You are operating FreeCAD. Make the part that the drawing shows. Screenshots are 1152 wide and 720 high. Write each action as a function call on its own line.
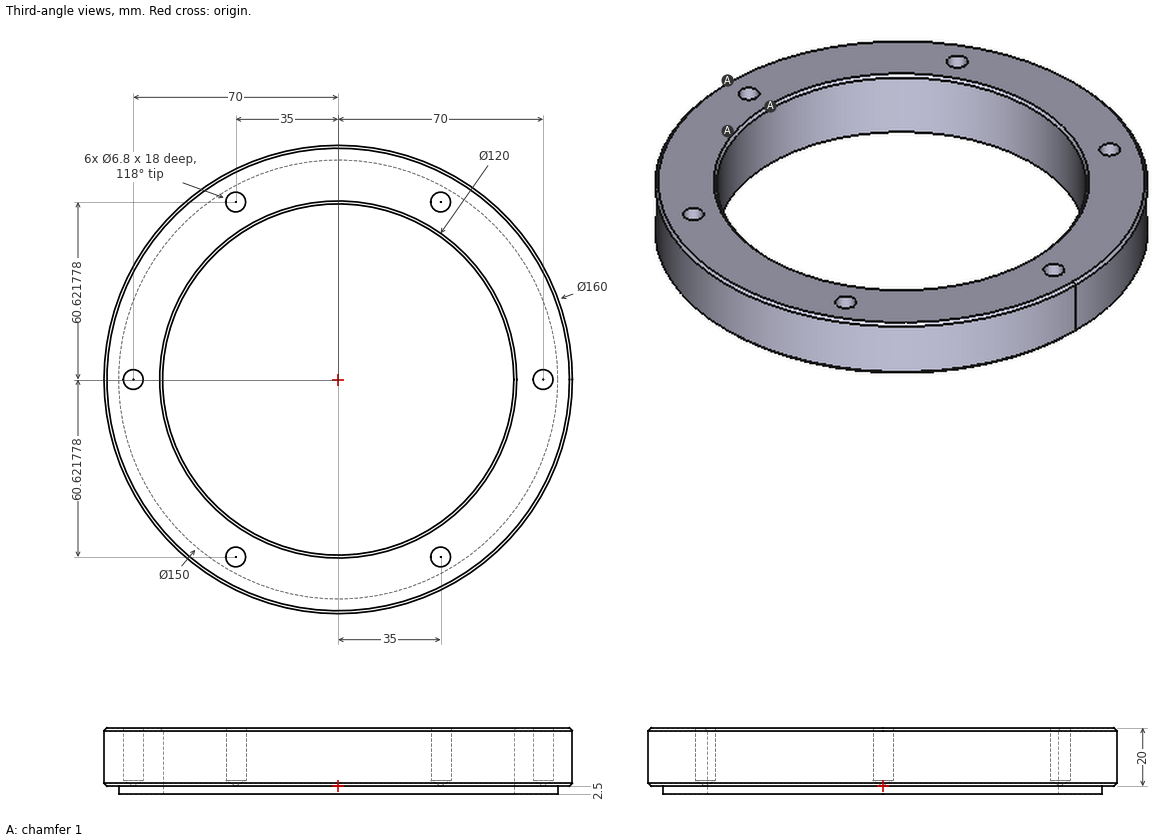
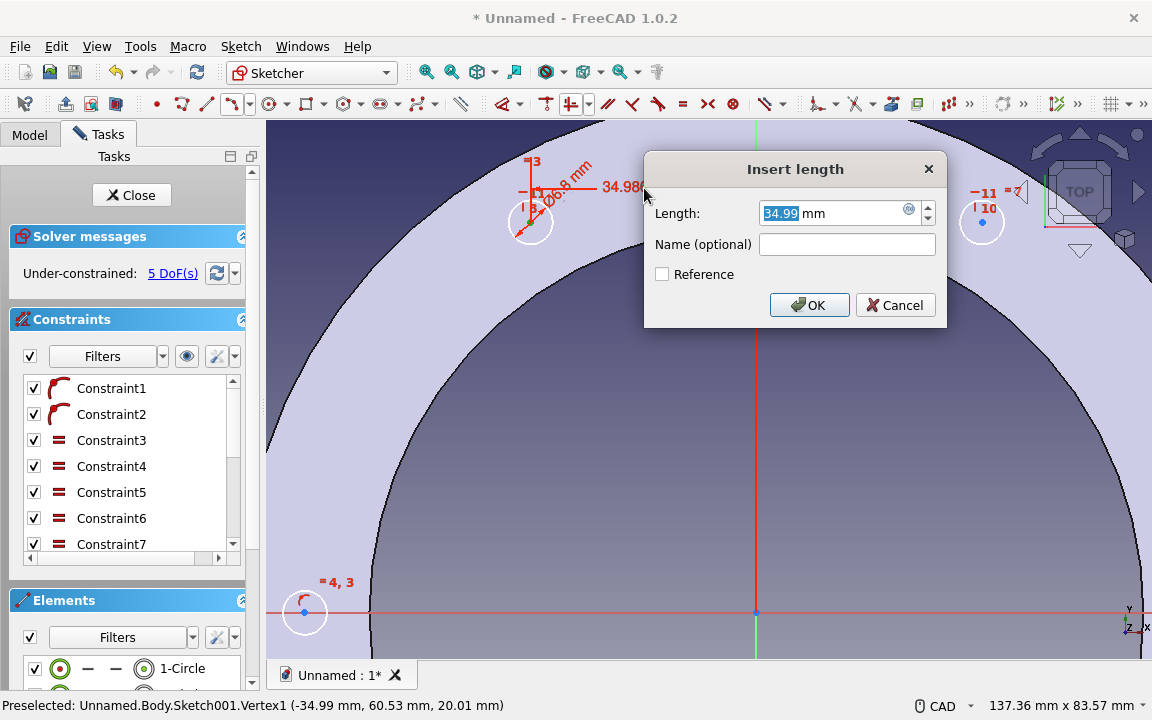
text(35)
key(Return)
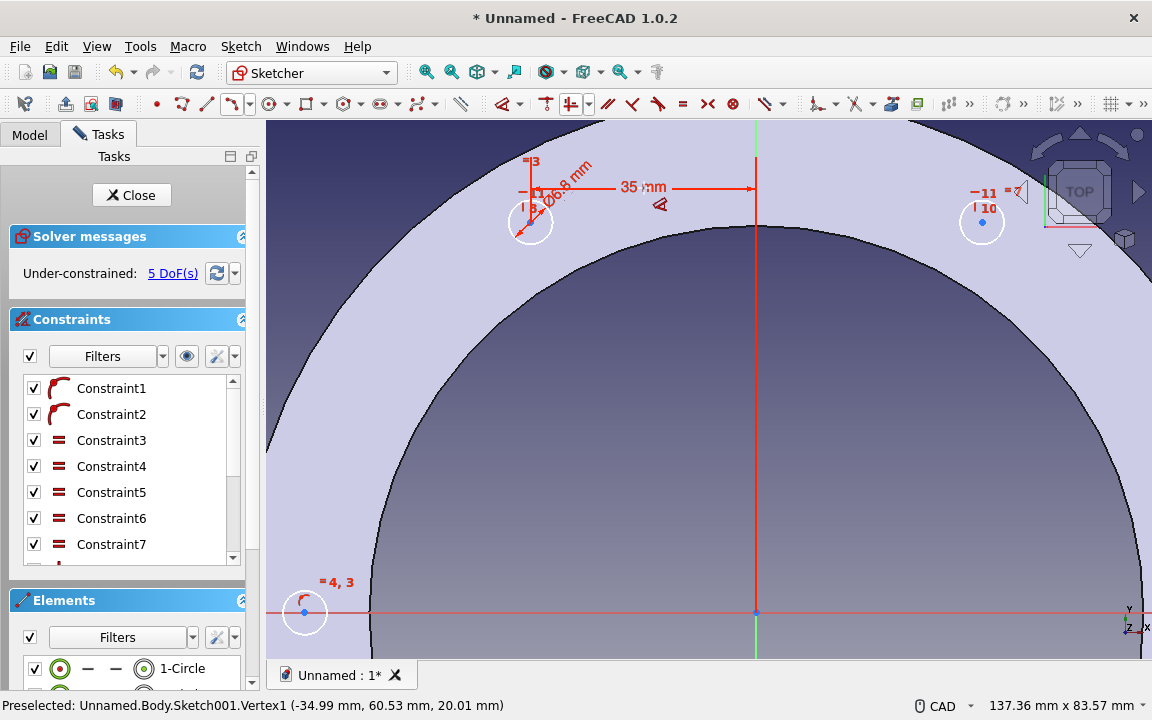
click(305, 613)
click(531, 579)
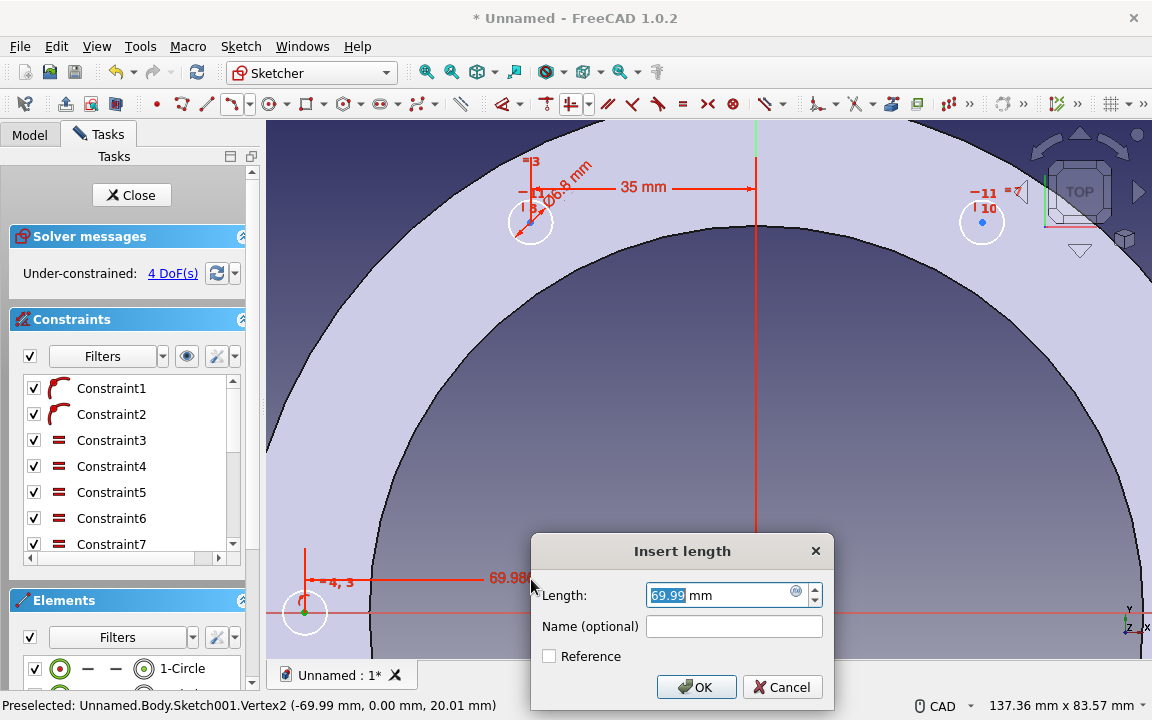
text(70)
key(Return)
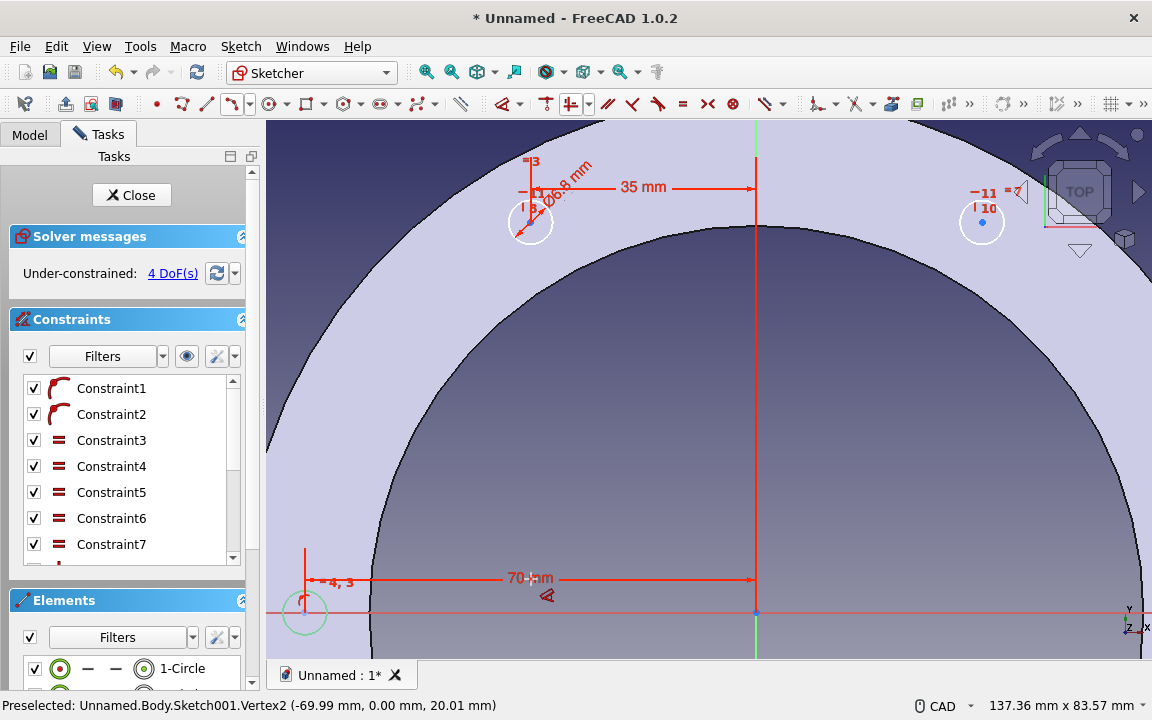
scroll(546, 207, down, 4)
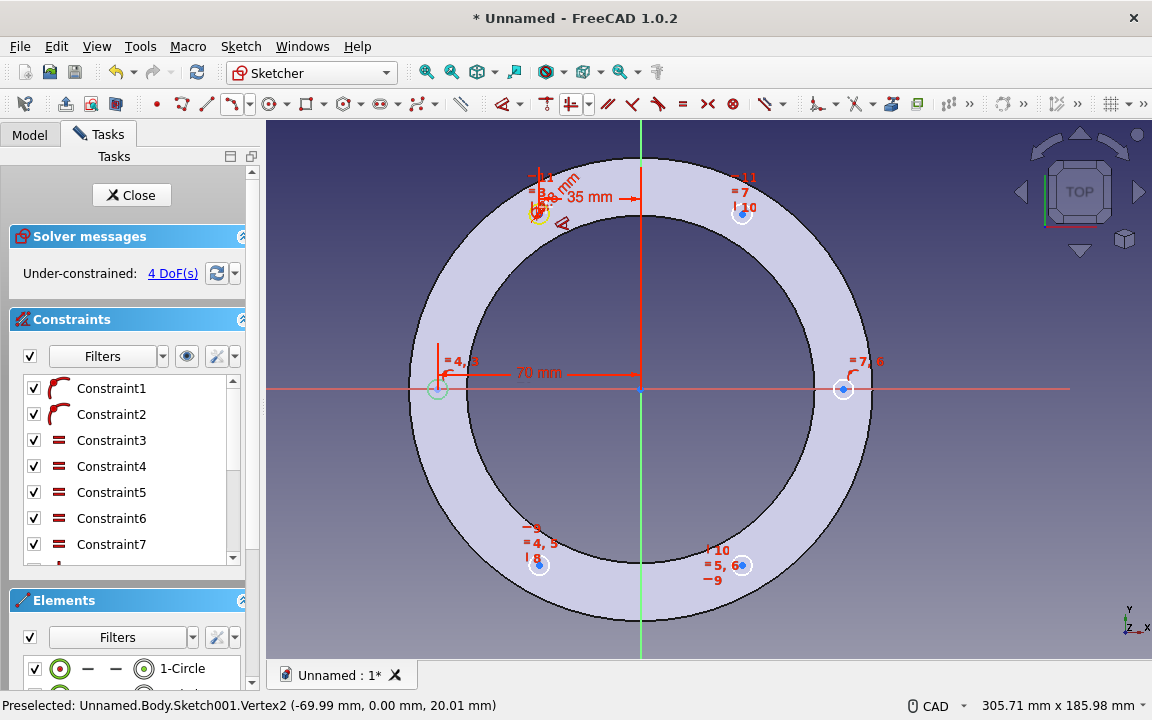
click(742, 565)
click(691, 599)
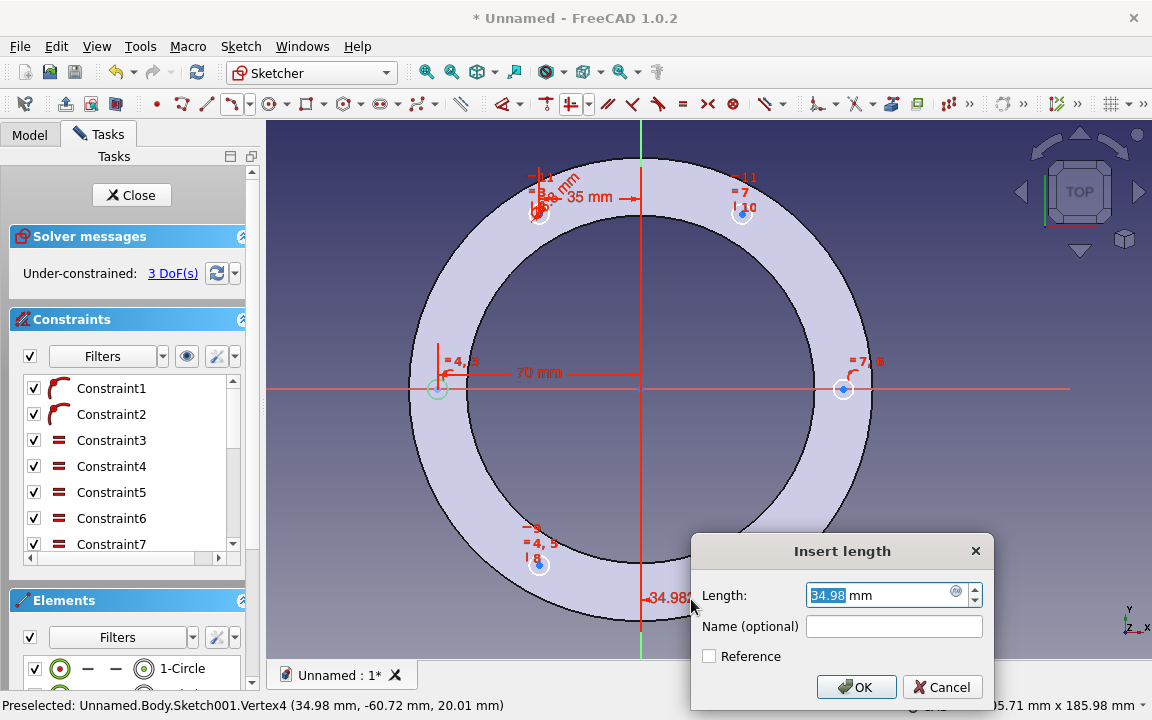
text(35)
key(Return)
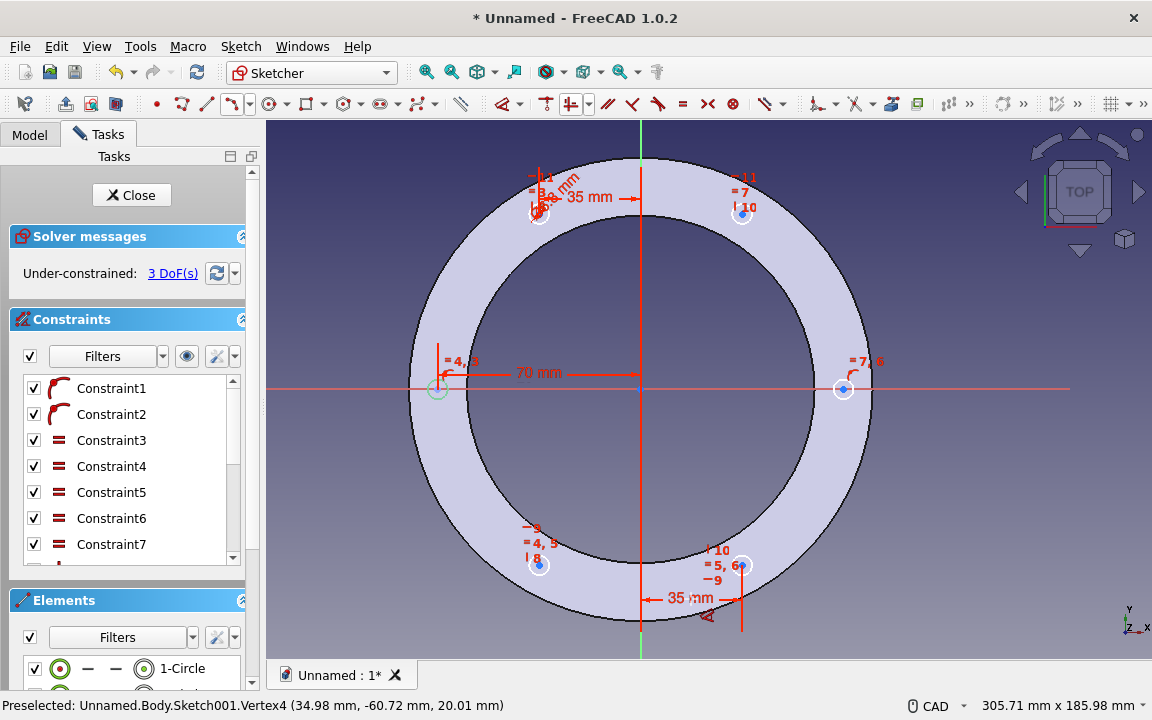
click(844, 389)
click(742, 423)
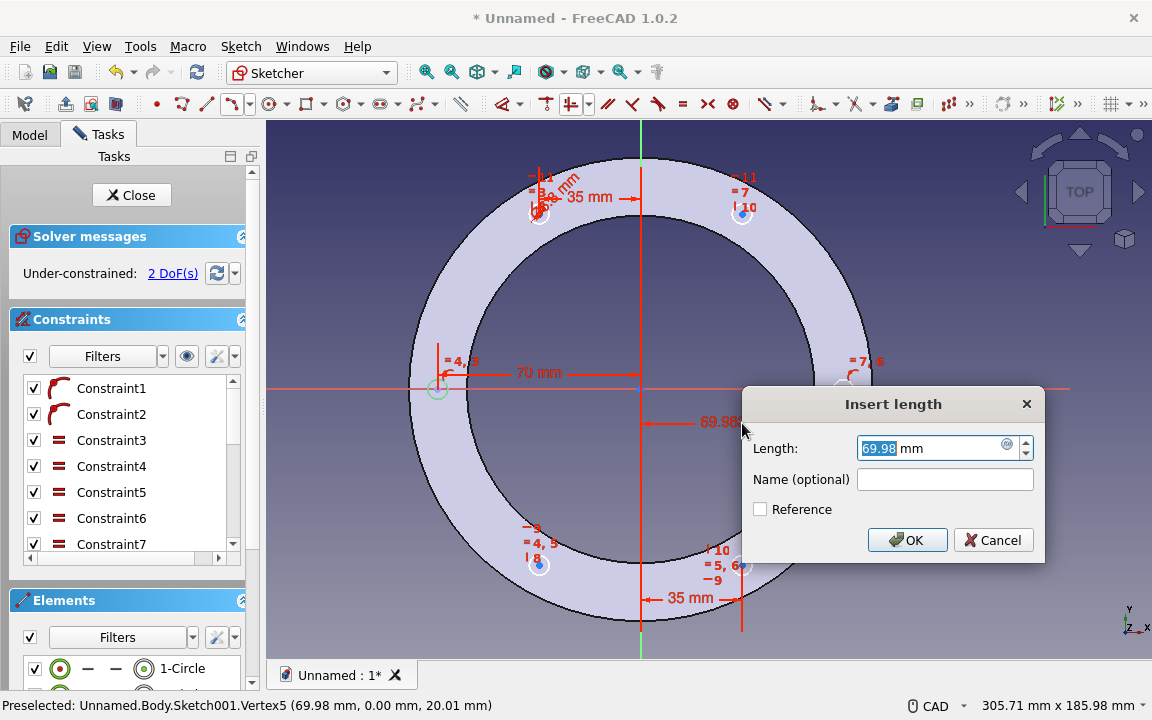
text(70)
key(Return)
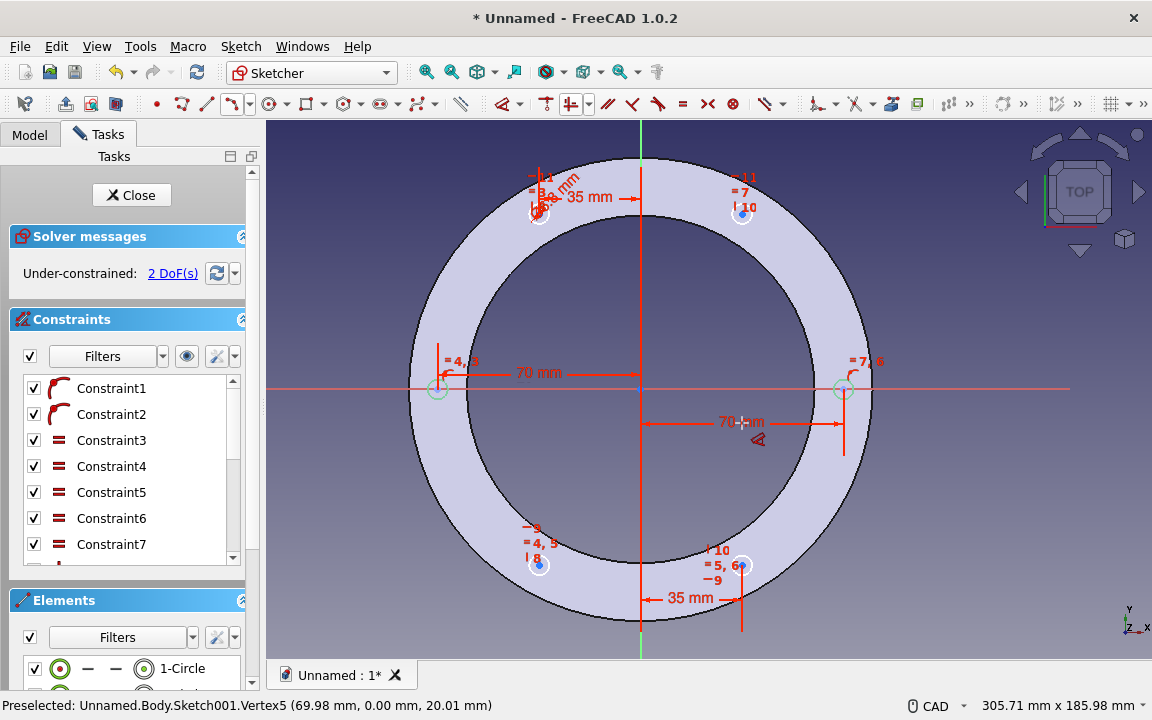
click(539, 214)
click(505, 302)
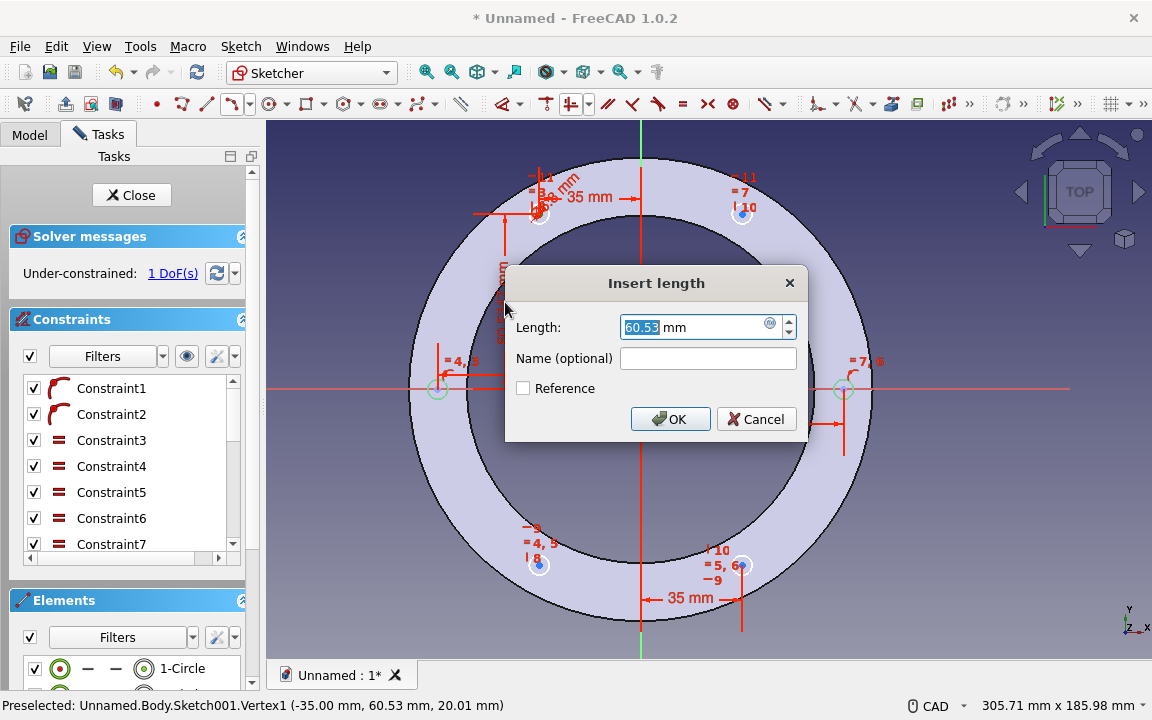
text(60.621778)
key(Return)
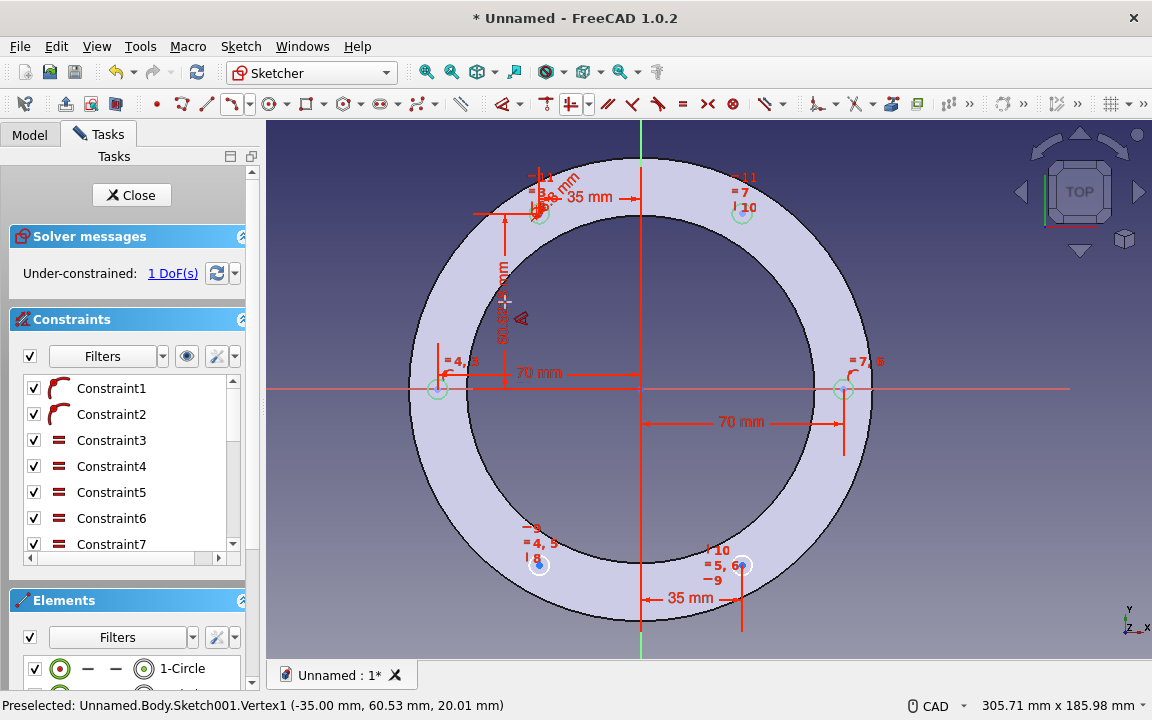
click(539, 565)
click(505, 477)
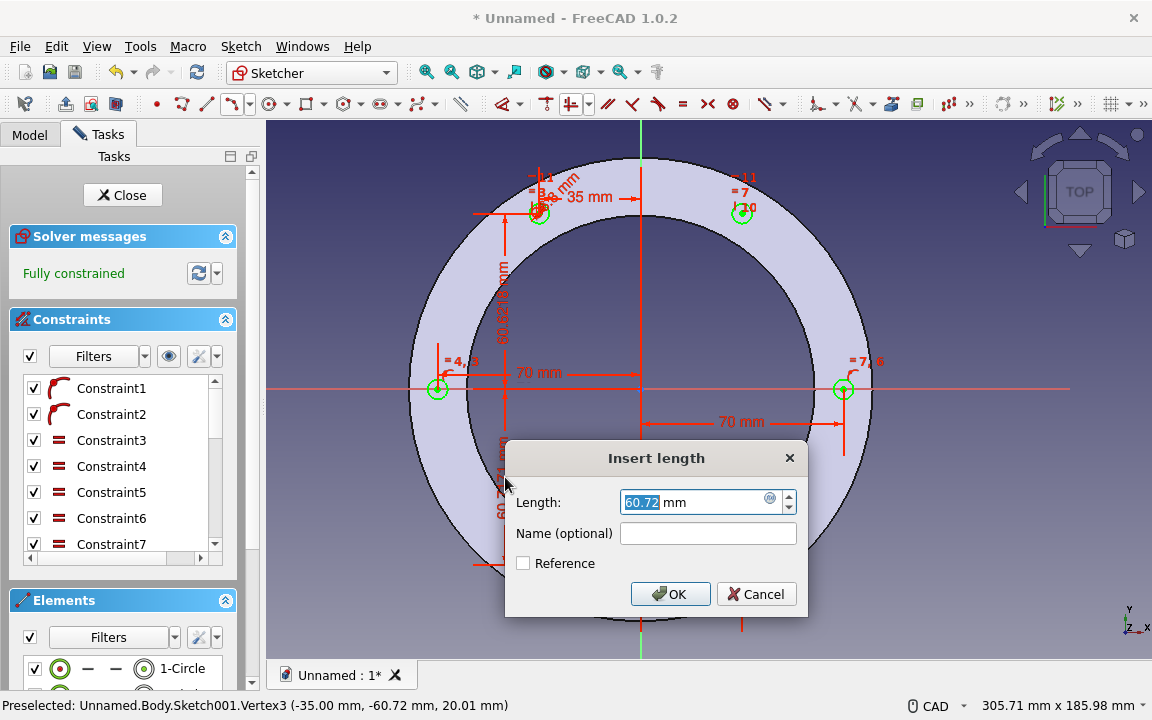
text(60.621778)
key(Return)
key(Escape)